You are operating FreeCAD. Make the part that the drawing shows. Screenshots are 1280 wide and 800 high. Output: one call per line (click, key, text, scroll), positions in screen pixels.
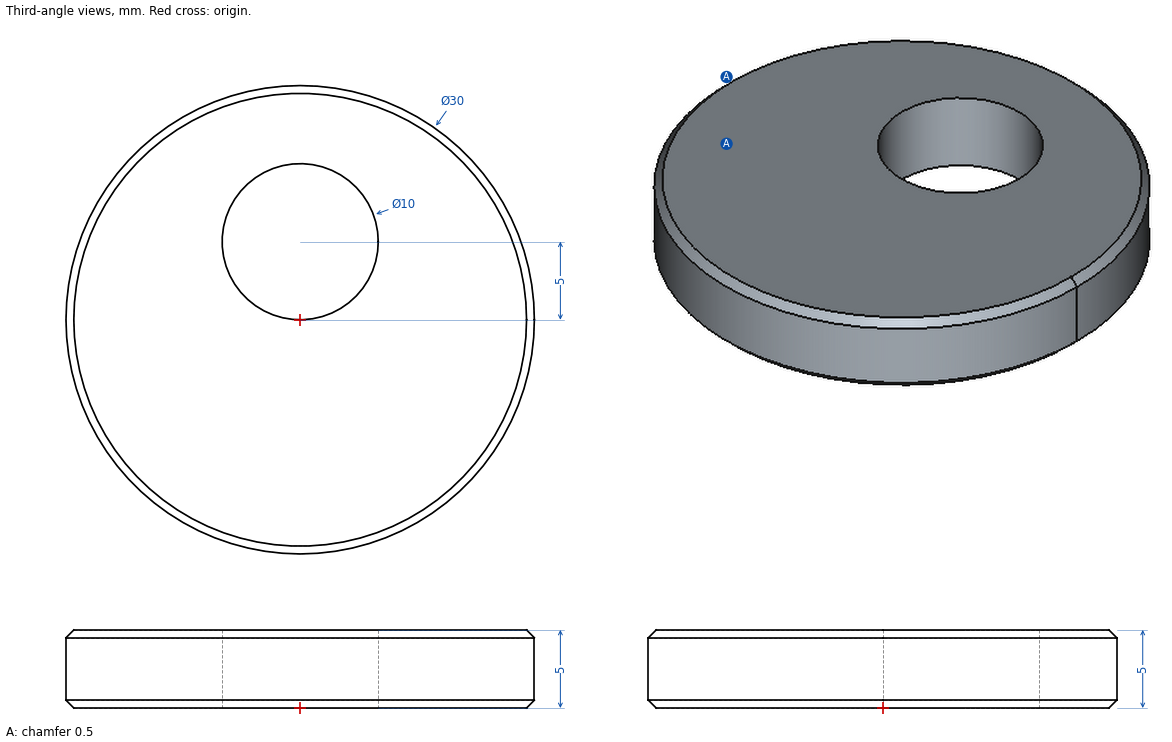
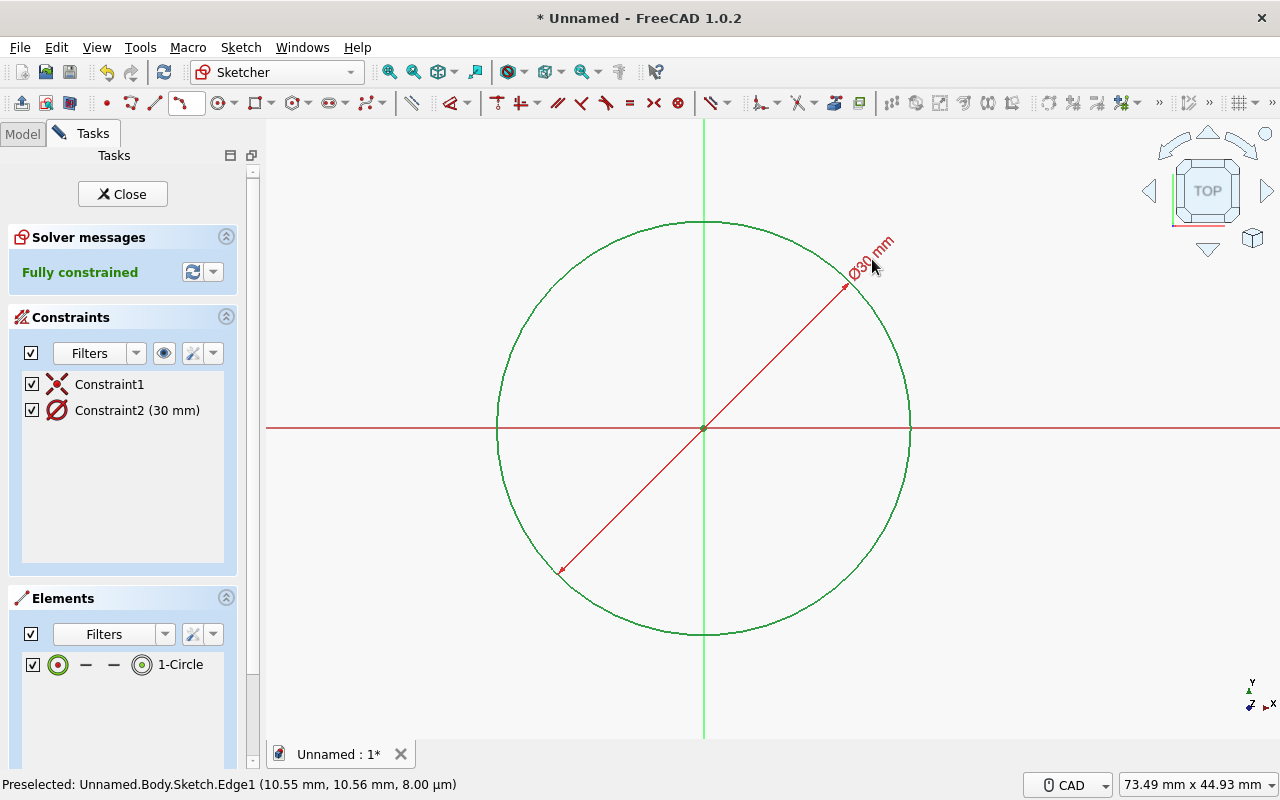
click(123, 194)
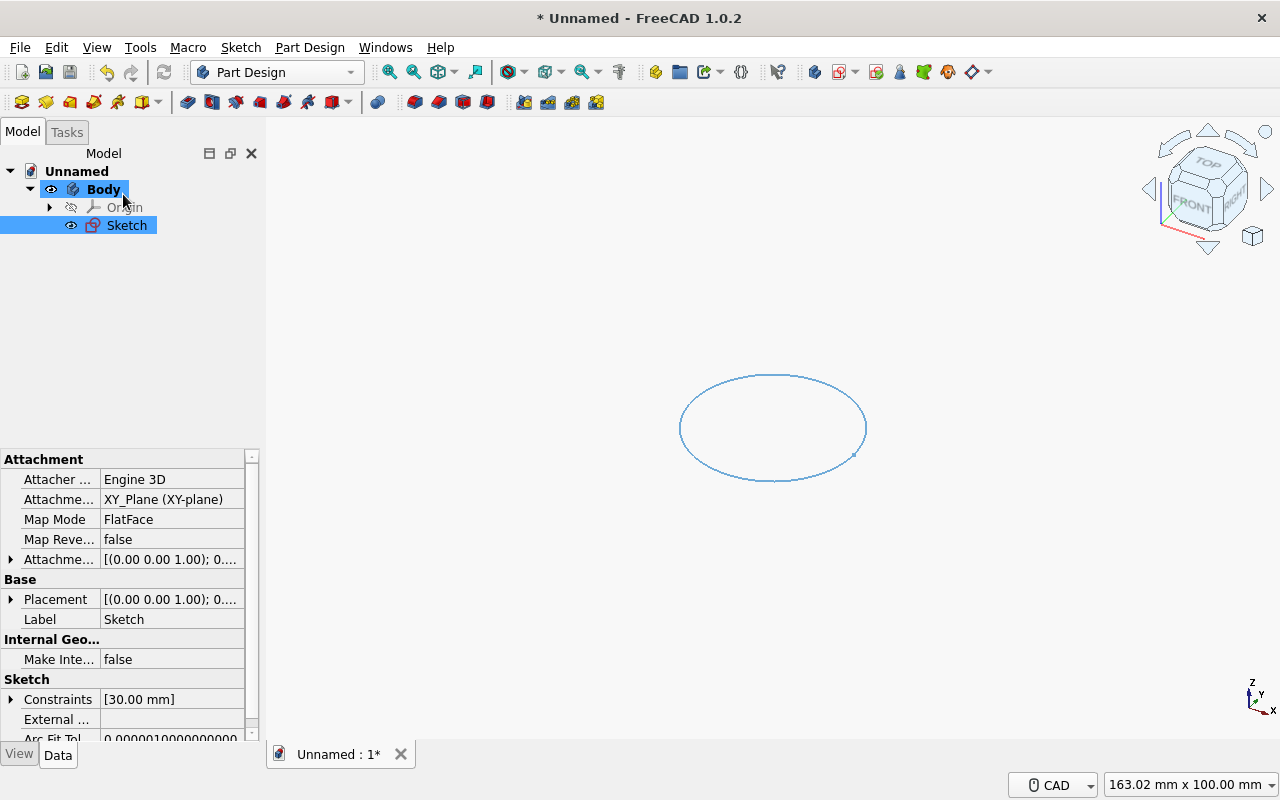
click(22, 102)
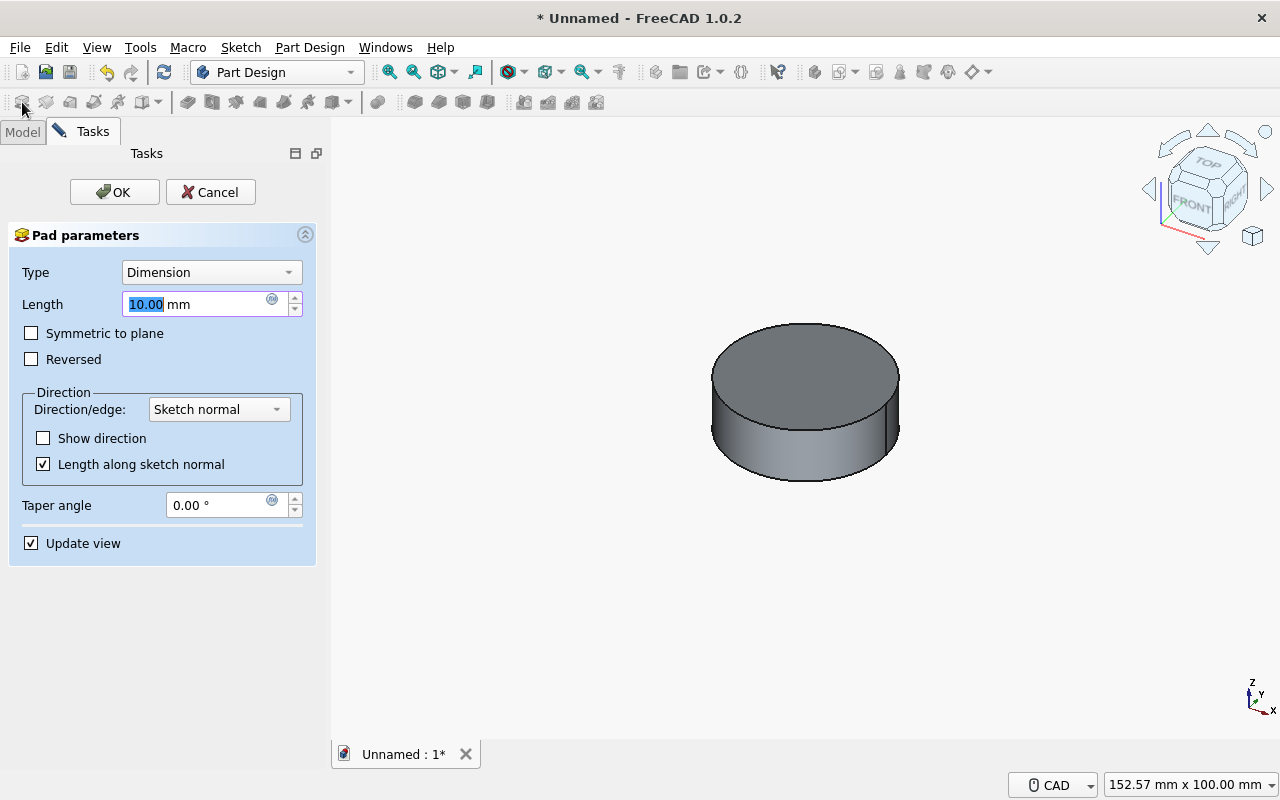
text(5)
key(Tab)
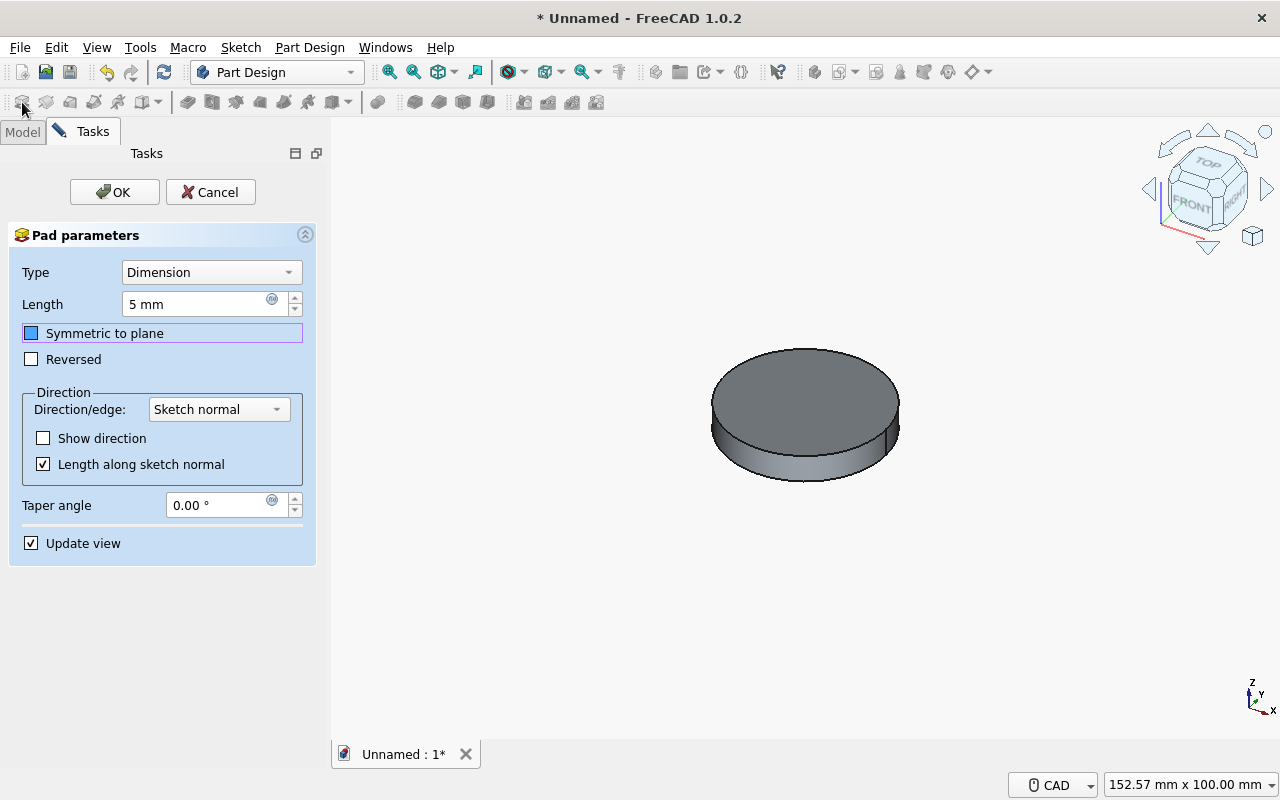
click(115, 192)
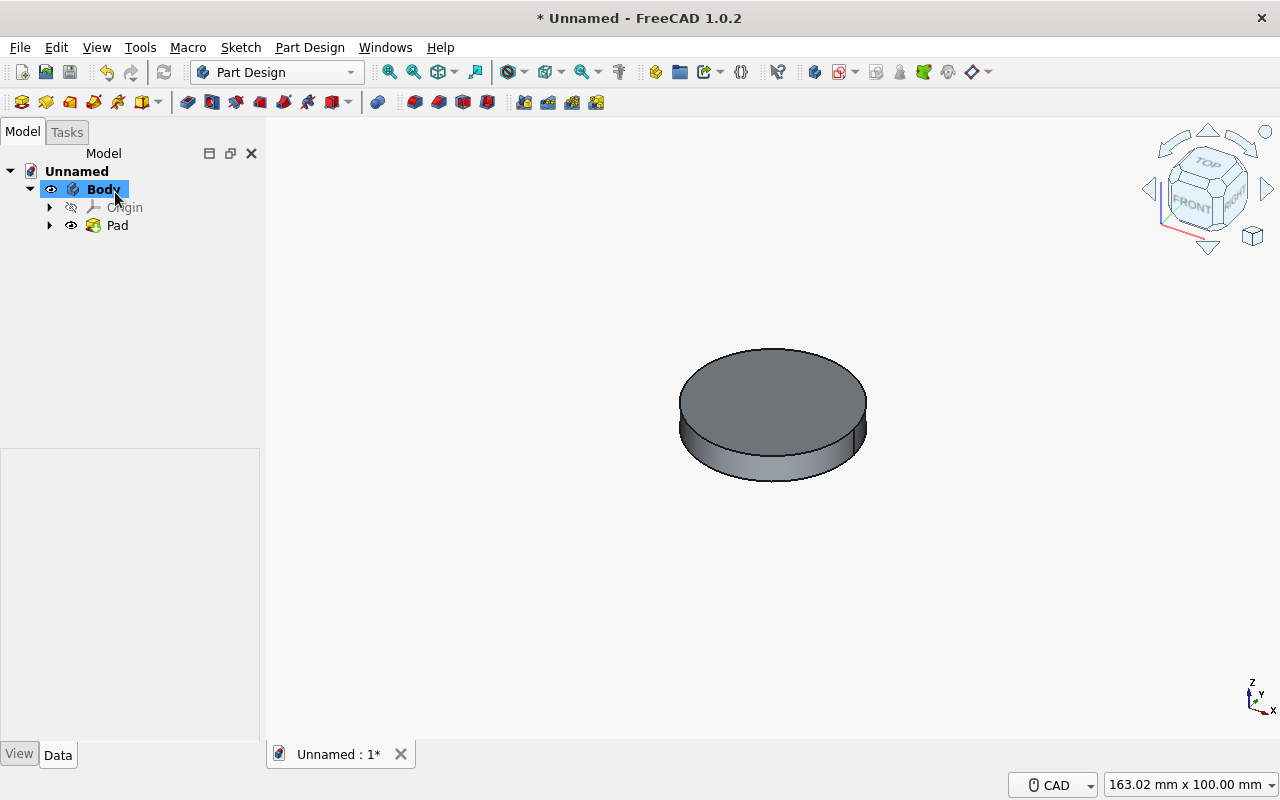
key(v)
key(f)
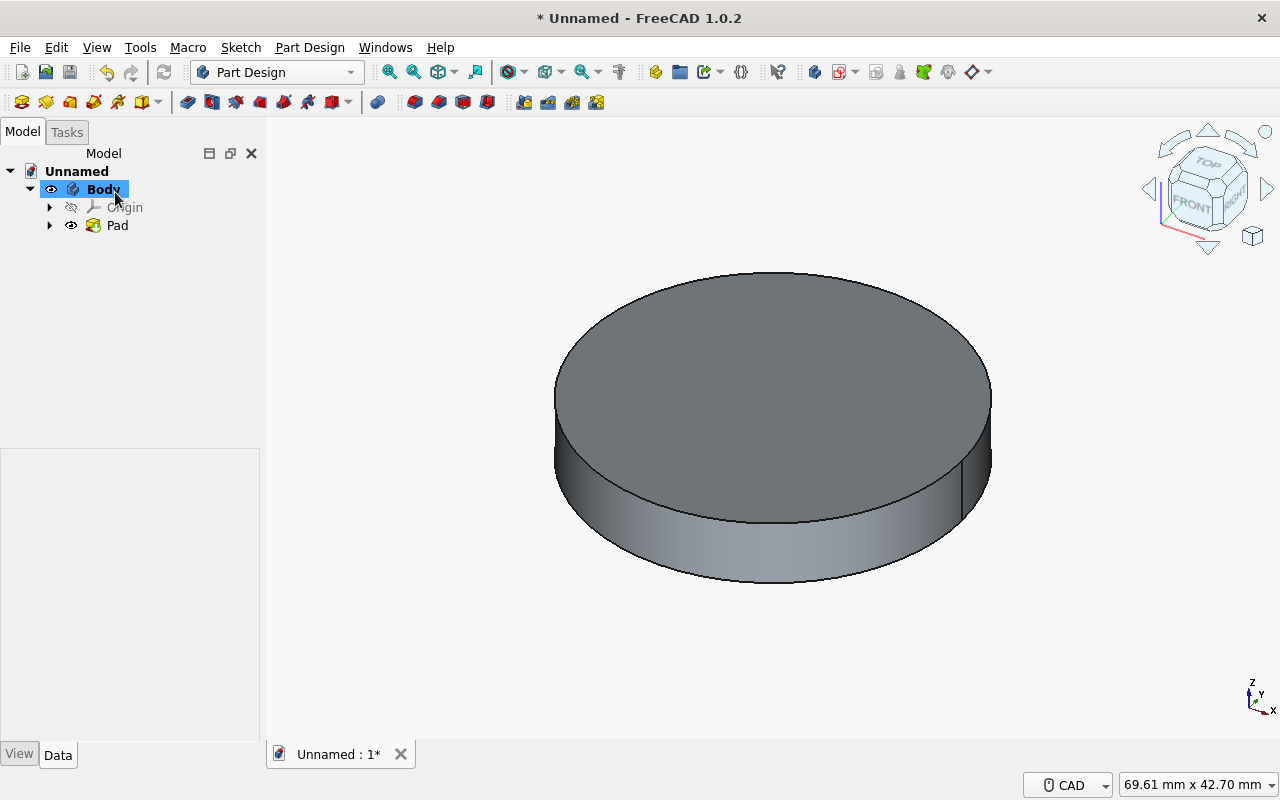
click(773, 397)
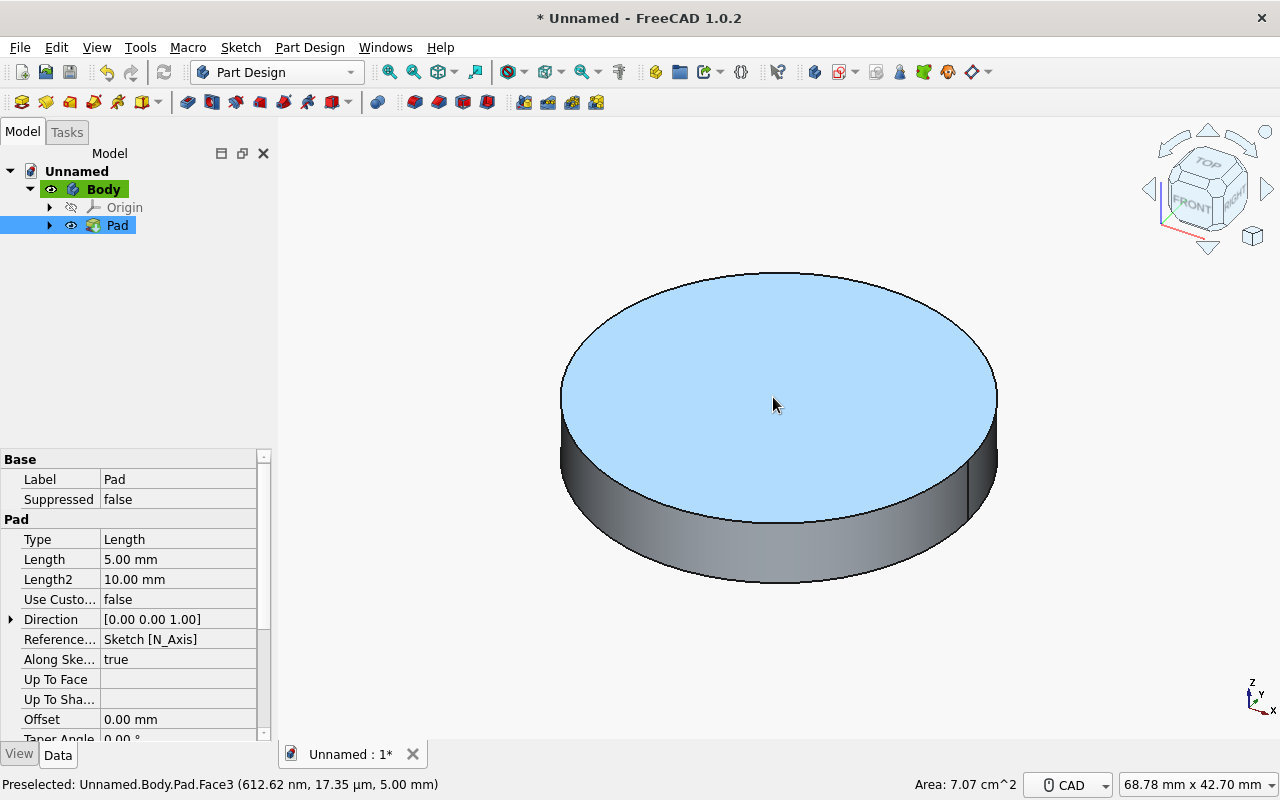
click(840, 72)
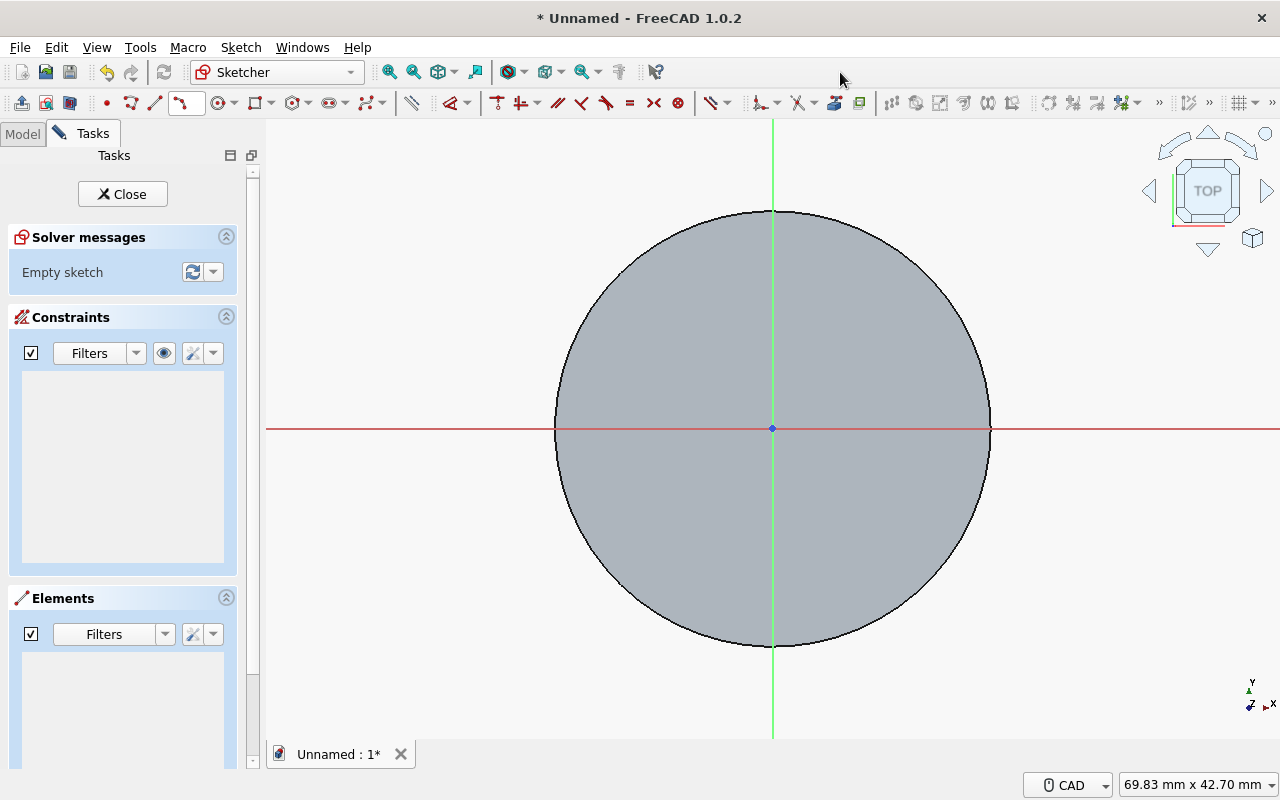
scroll(813, 314, up, 5)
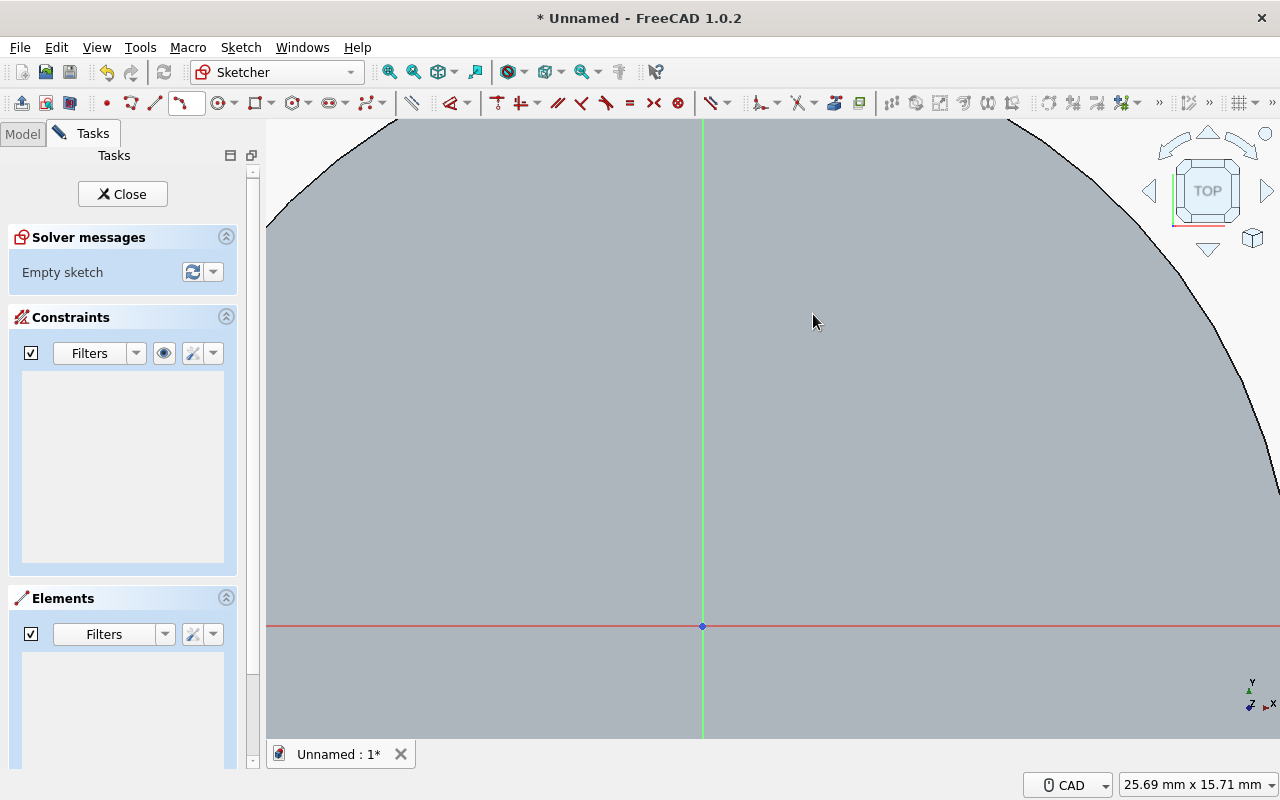
key(g)
key(c)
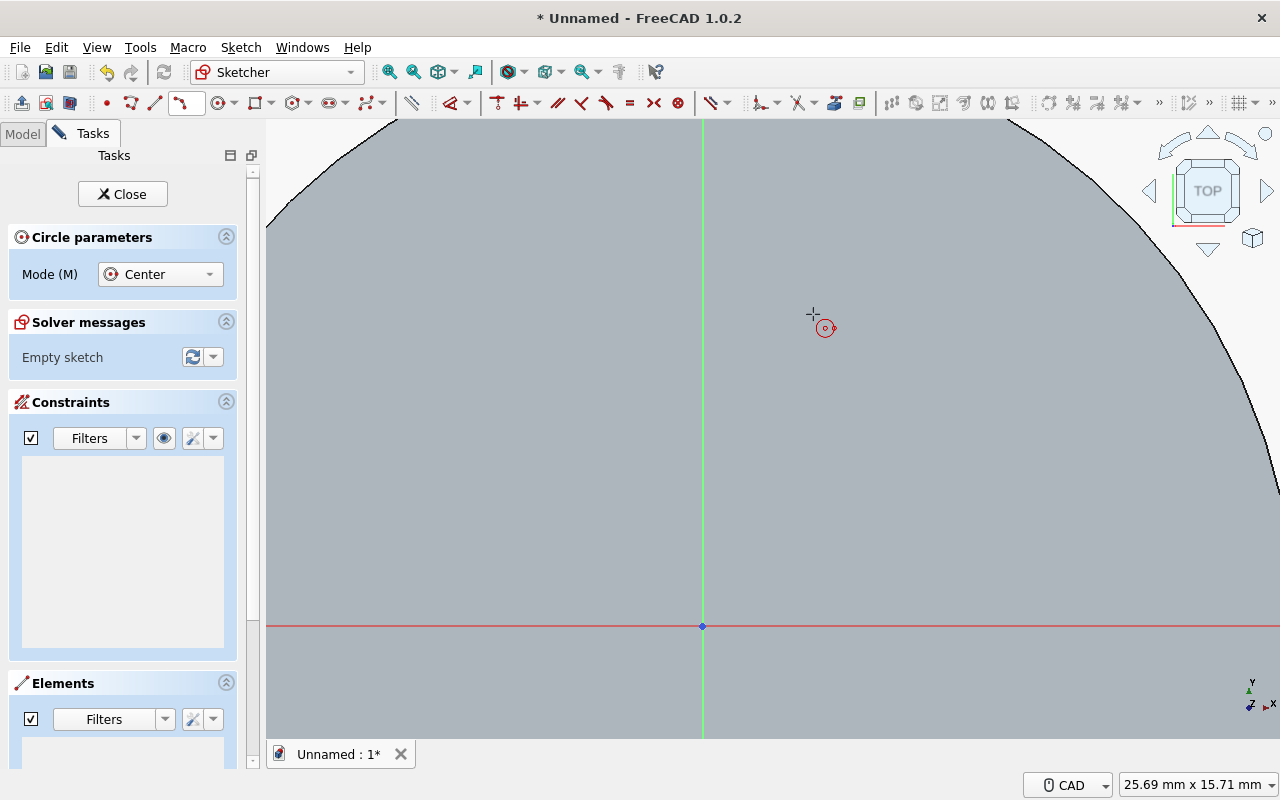
click(703, 429)
click(842, 289)
key(Escape)